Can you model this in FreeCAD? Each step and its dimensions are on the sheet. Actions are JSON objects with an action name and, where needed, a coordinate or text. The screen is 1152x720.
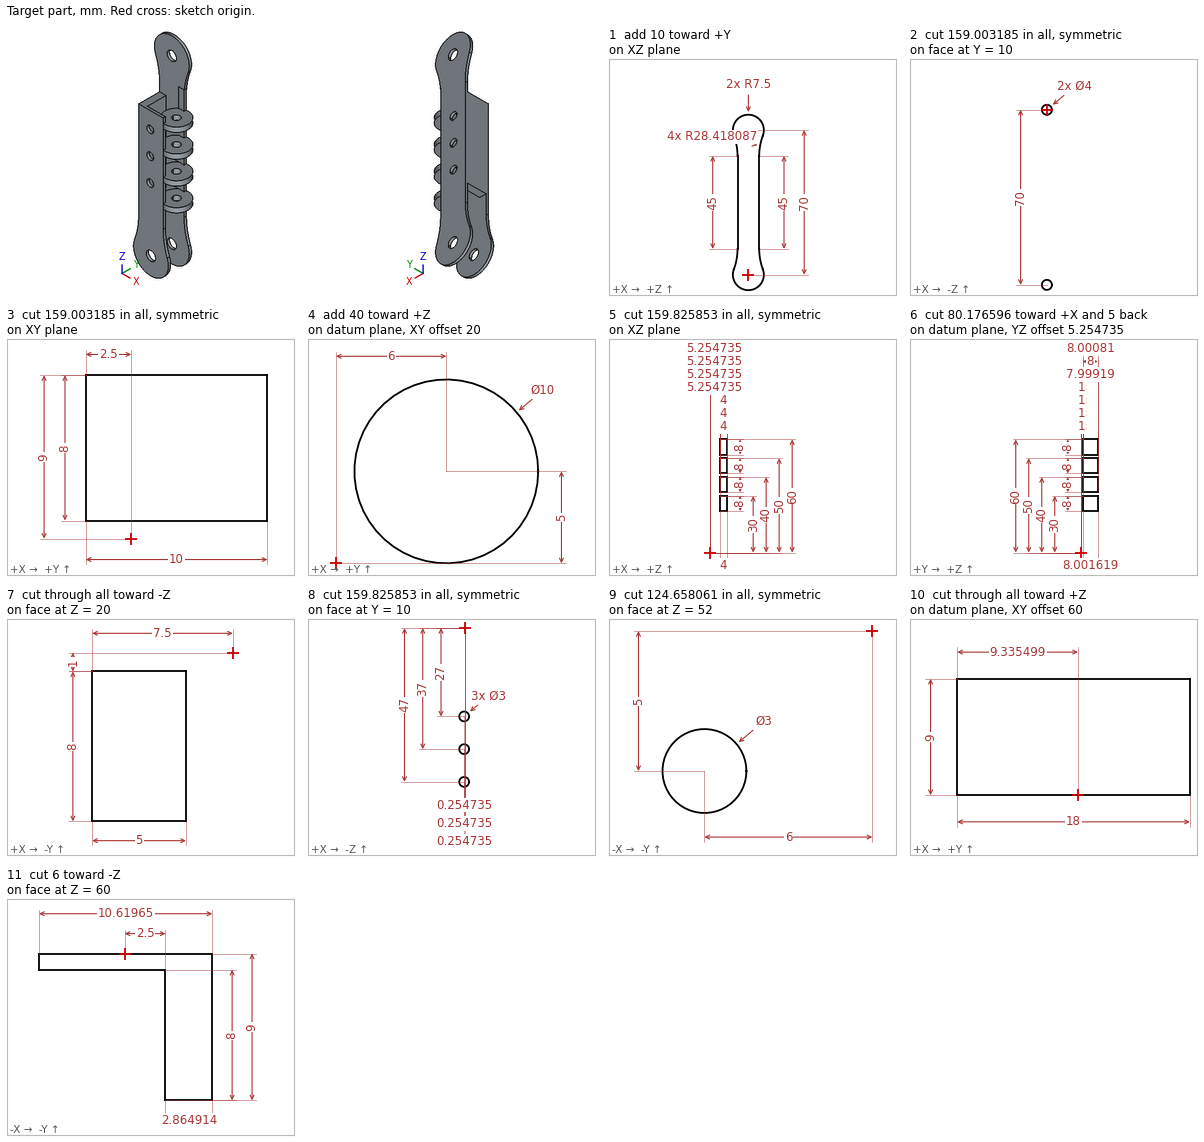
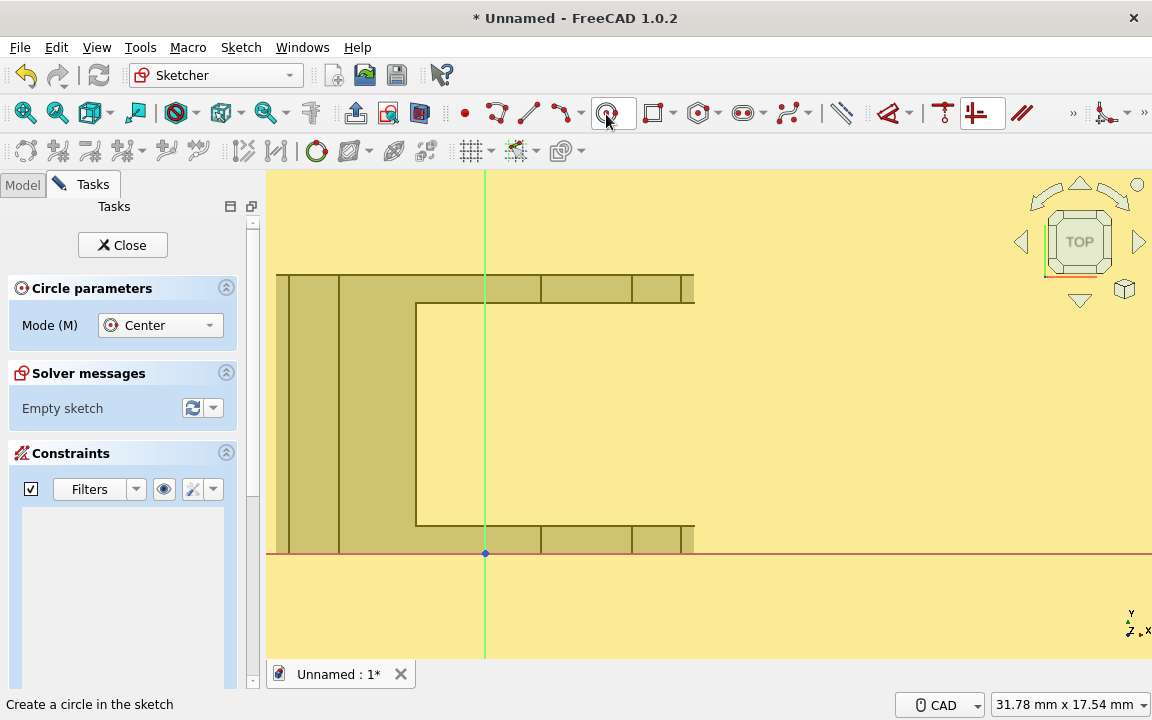
{"action": "left_click", "coordinate": [653, 414]}
{"action": "left_click", "coordinate": [751, 316]}
{"action": "key", "text": "Escape"}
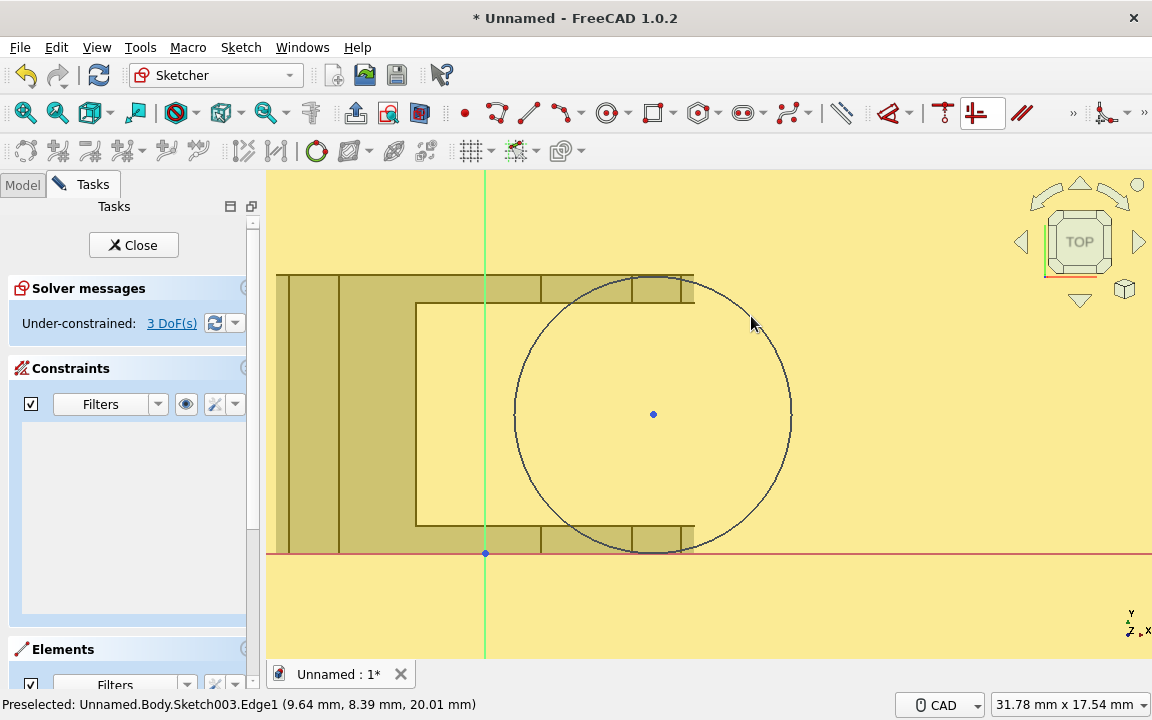
{"action": "left_click", "coordinate": [888, 114]}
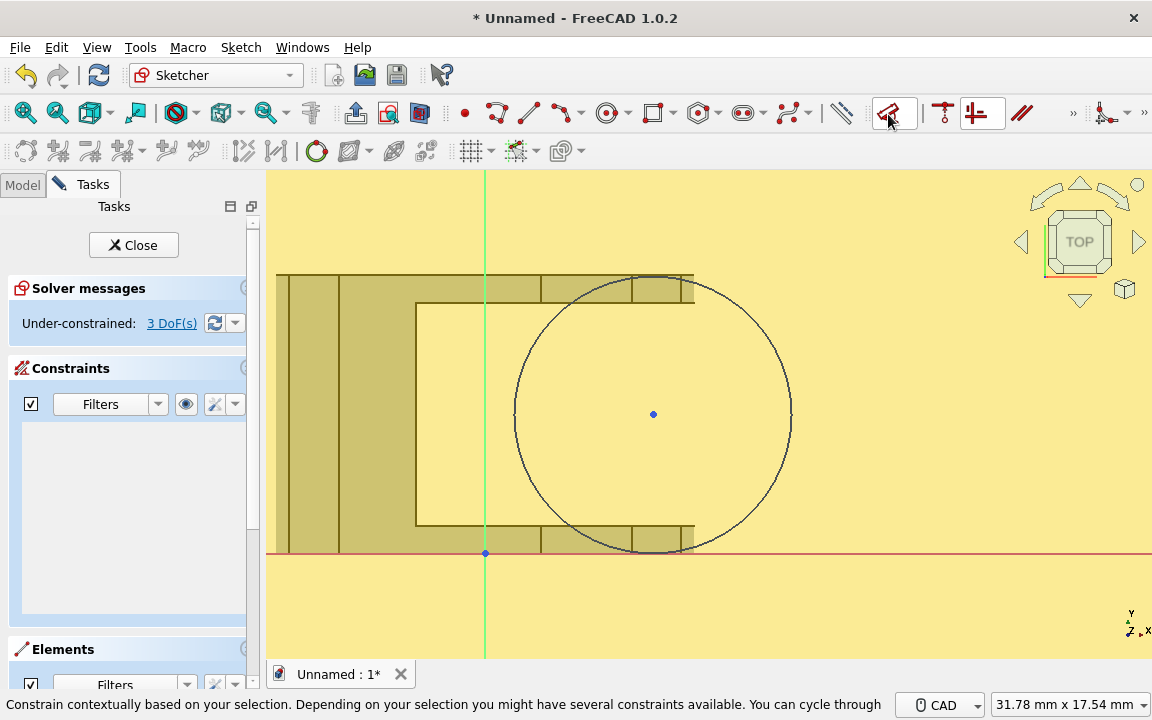
{"action": "left_click", "coordinate": [751, 317]}
{"action": "left_click", "coordinate": [774, 294]}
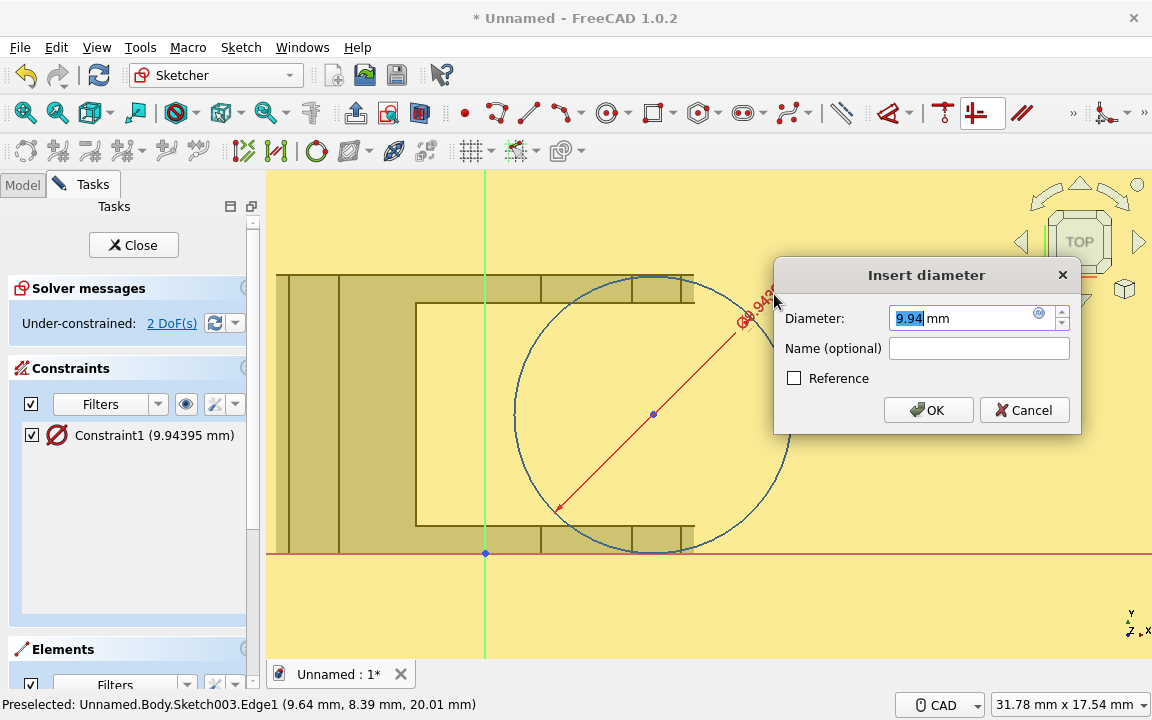
{"action": "type", "text": "10"}
{"action": "key", "text": "Return"}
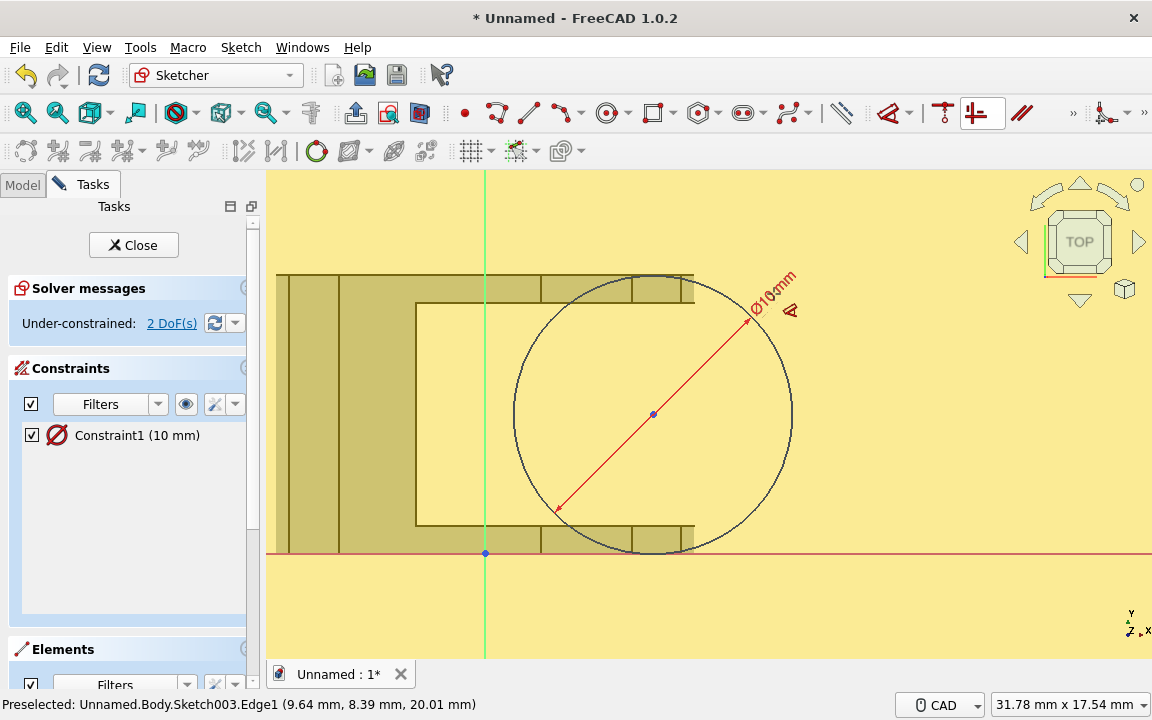
{"action": "left_click", "coordinate": [653, 415]}
{"action": "left_click", "coordinate": [569, 588]}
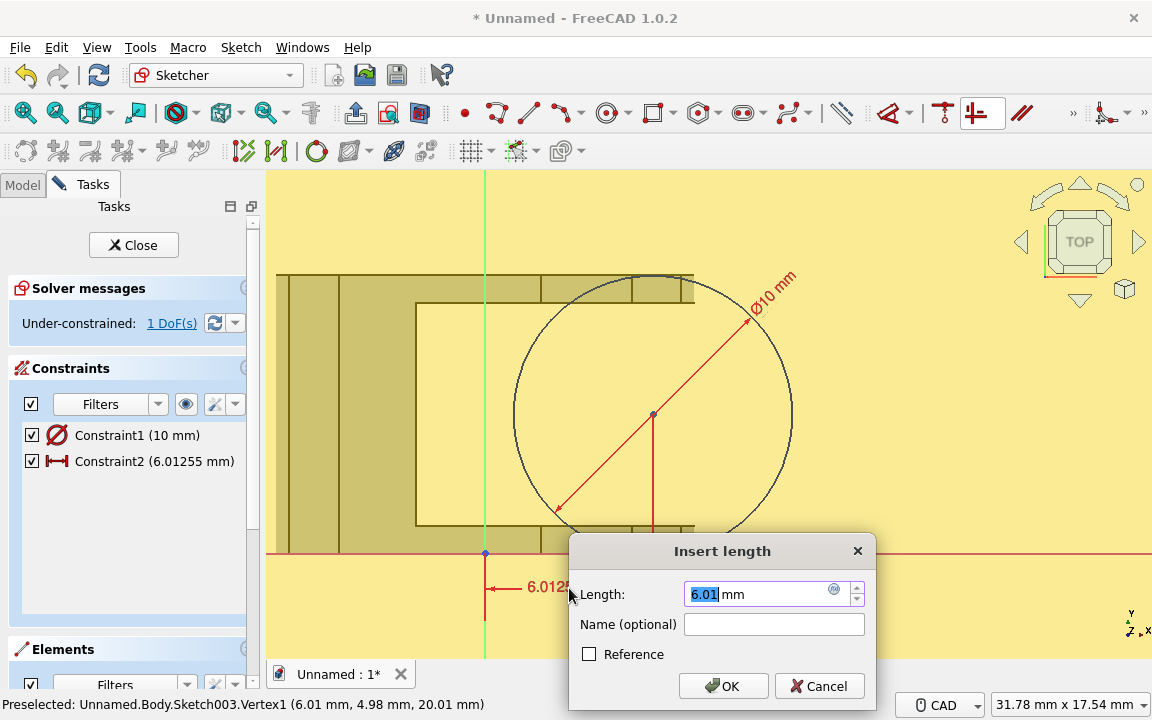
{"action": "type", "text": "6"}
{"action": "key", "text": "Return"}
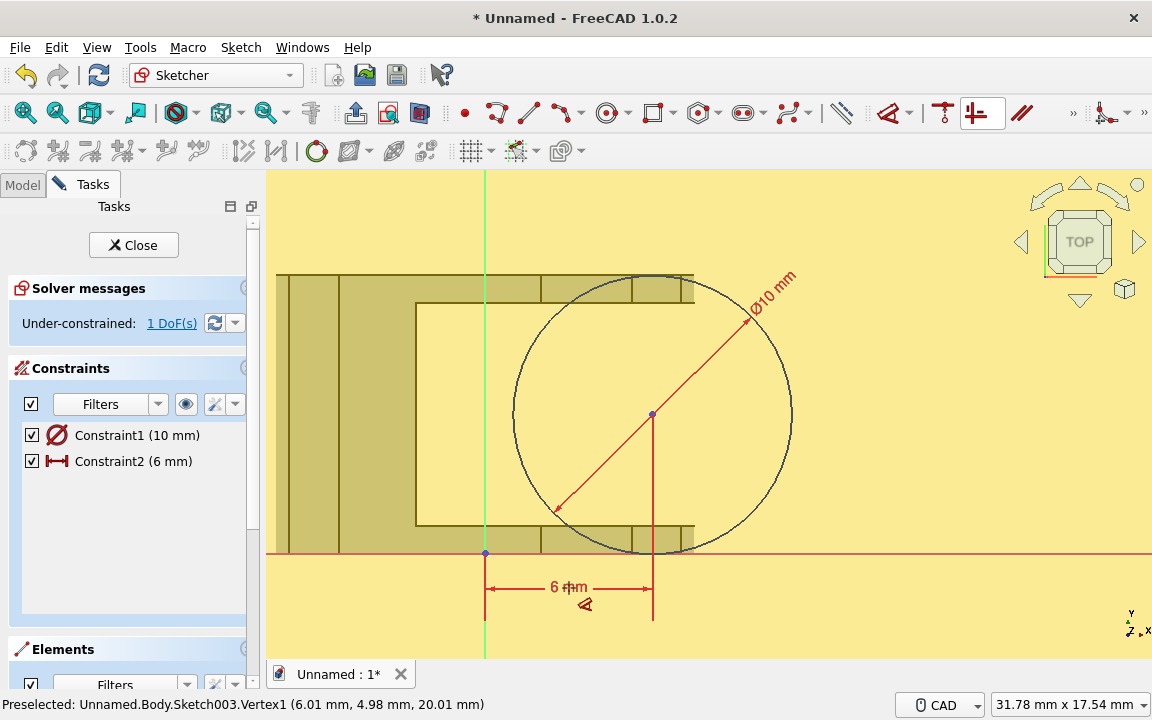
{"action": "left_click", "coordinate": [653, 415]}
{"action": "left_click", "coordinate": [451, 484]}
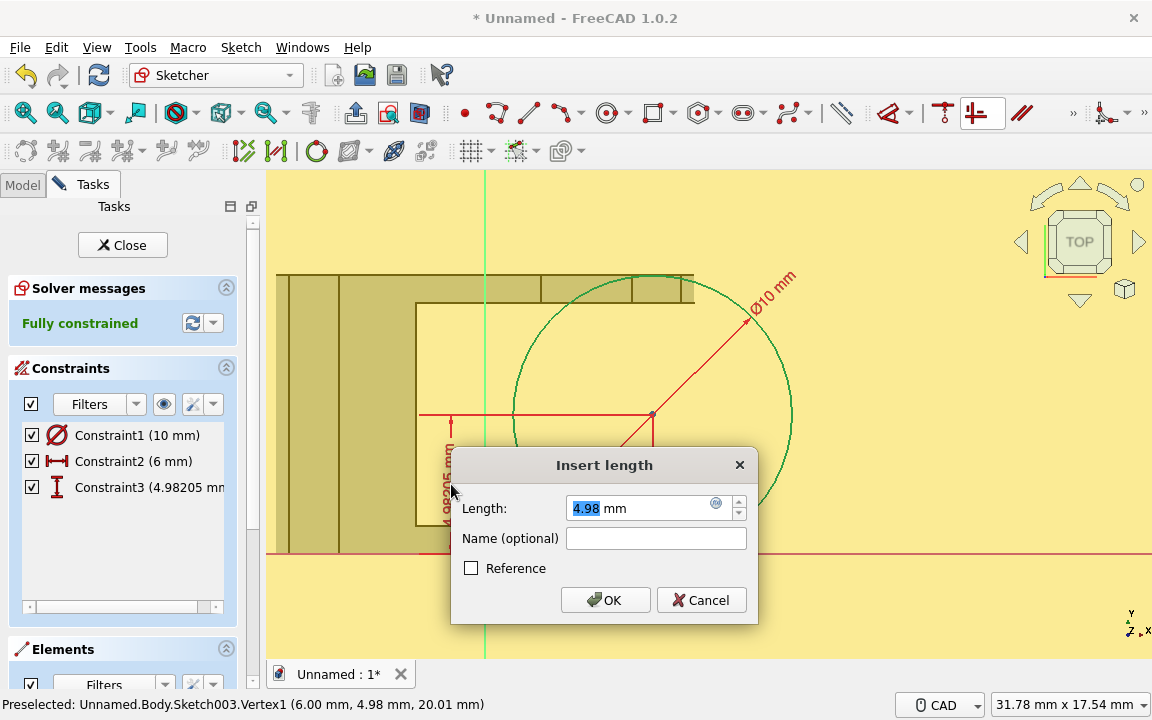
{"action": "type", "text": "5"}
{"action": "key", "text": "Return"}
{"action": "key", "text": "Escape"}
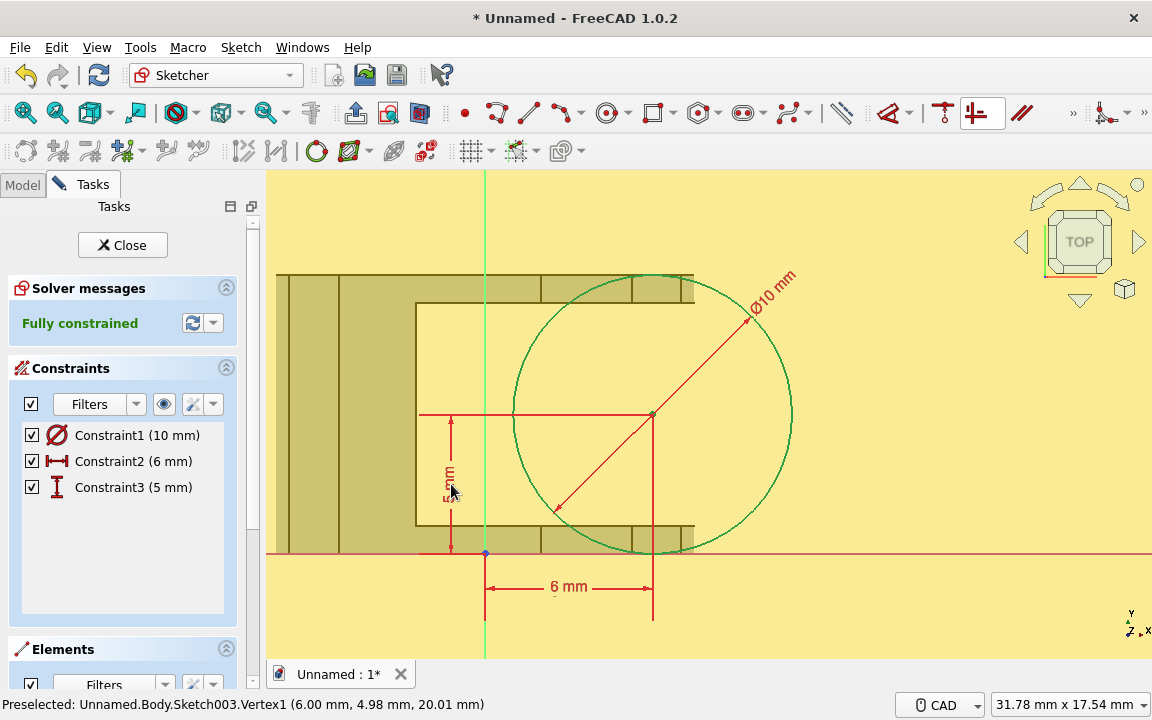
{"action": "left_click", "coordinate": [123, 245]}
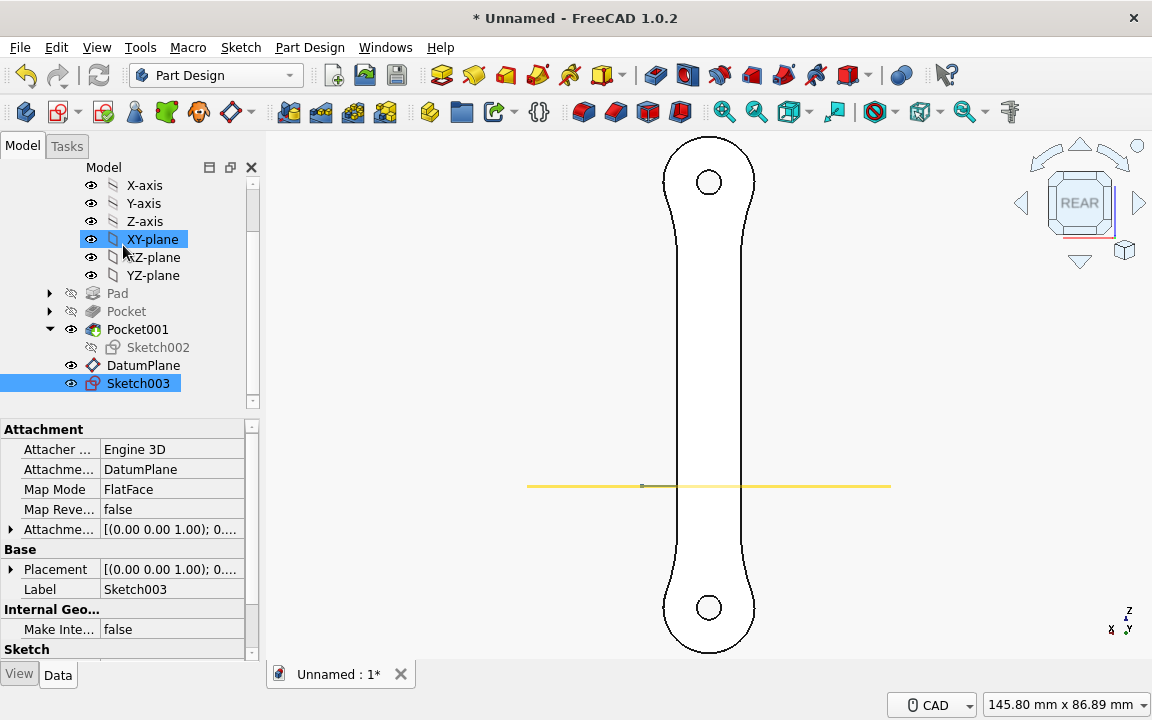
{"action": "left_click", "coordinate": [442, 76]}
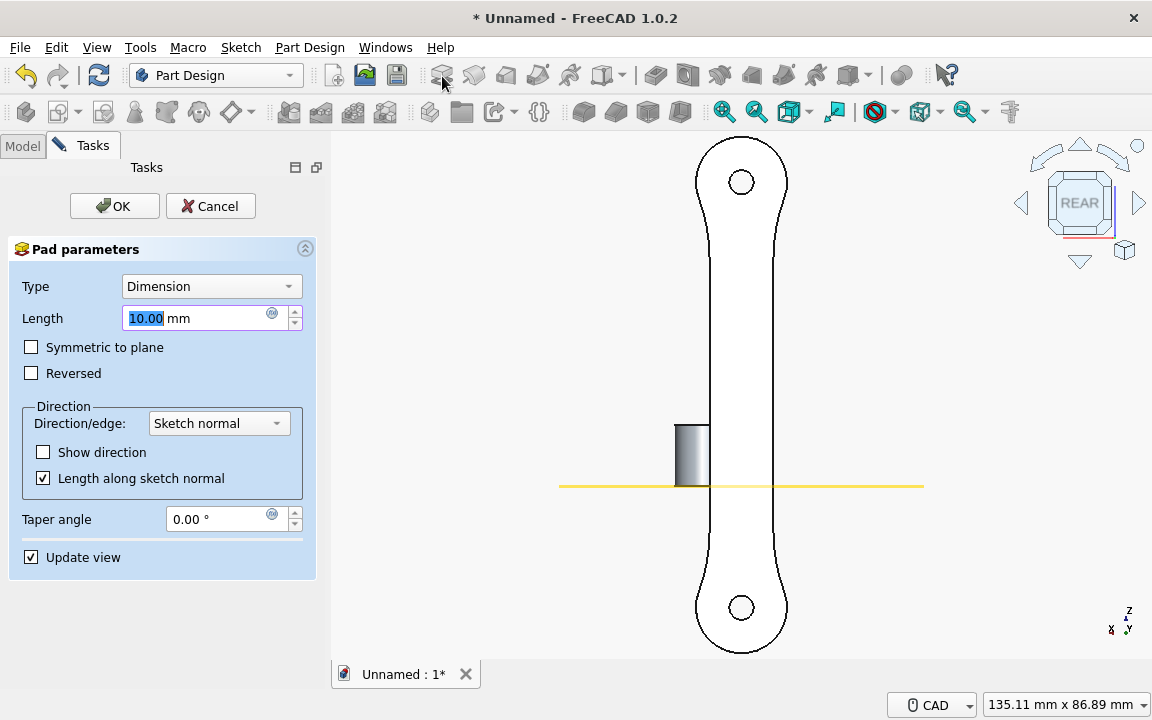
{"action": "type", "text": "40"}
{"action": "key", "text": "Tab"}